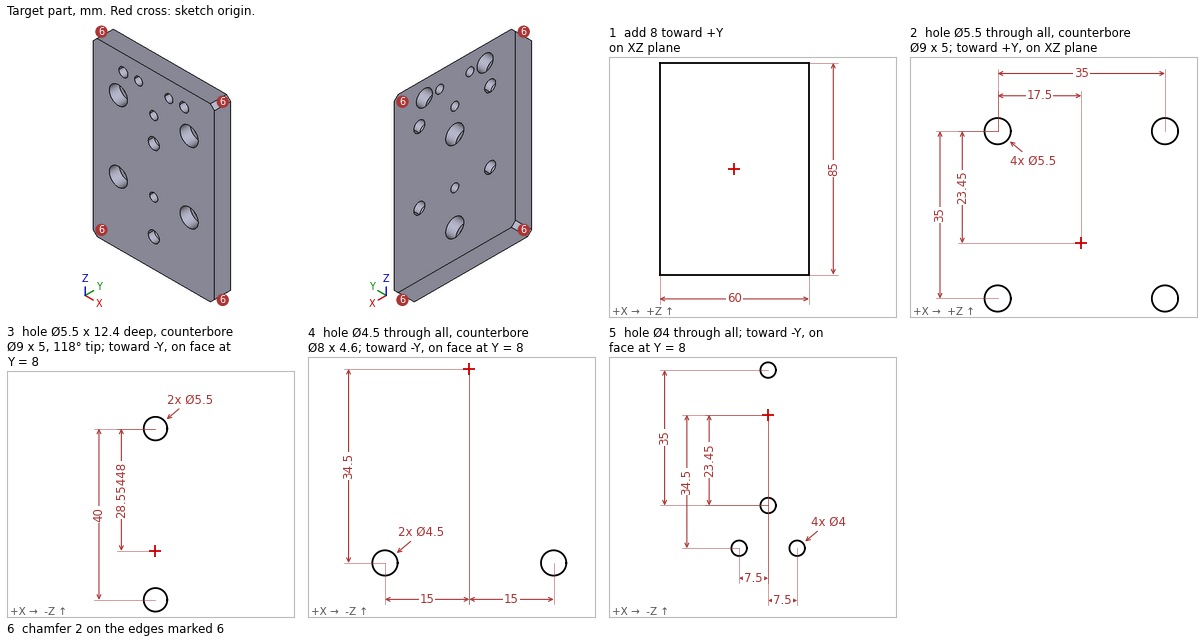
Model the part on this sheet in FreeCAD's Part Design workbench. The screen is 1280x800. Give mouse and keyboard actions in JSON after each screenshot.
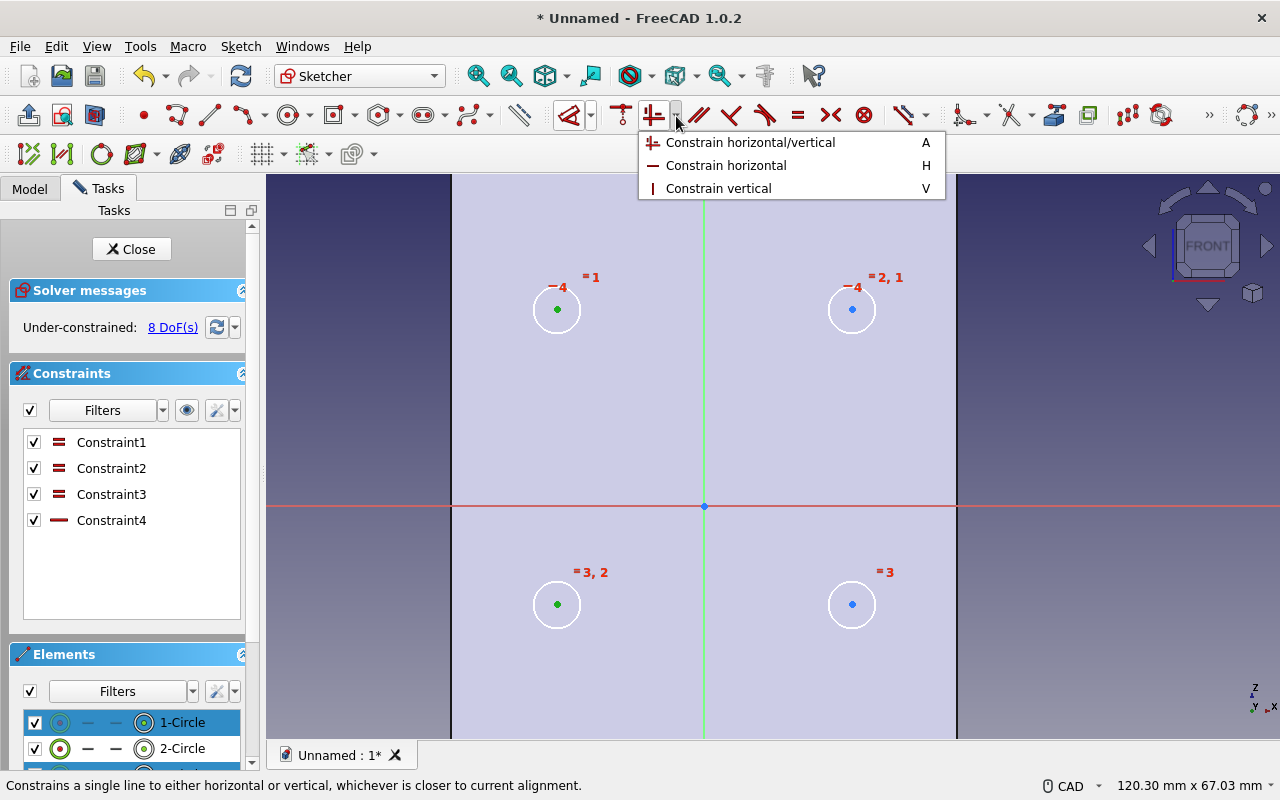
{"action": "left_click", "coordinate": [792, 188]}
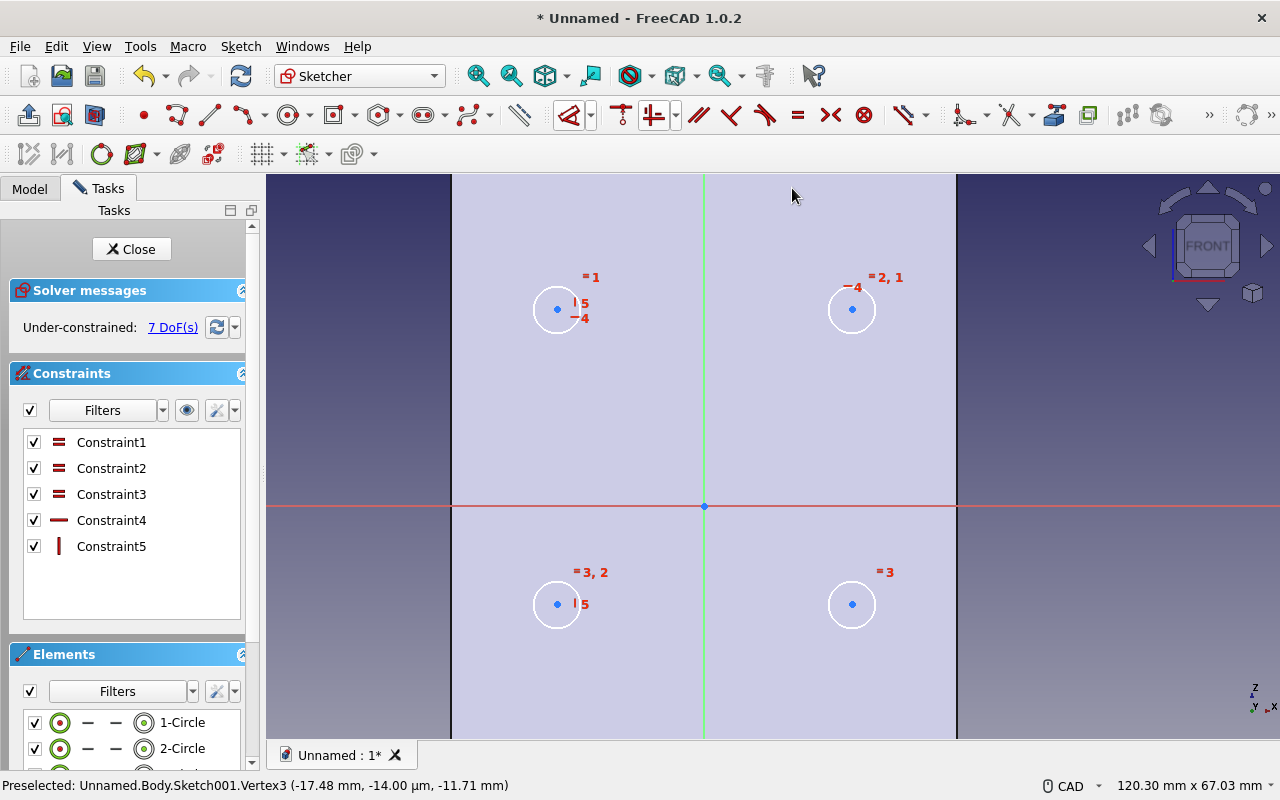
{"action": "left_click", "coordinate": [852, 310]}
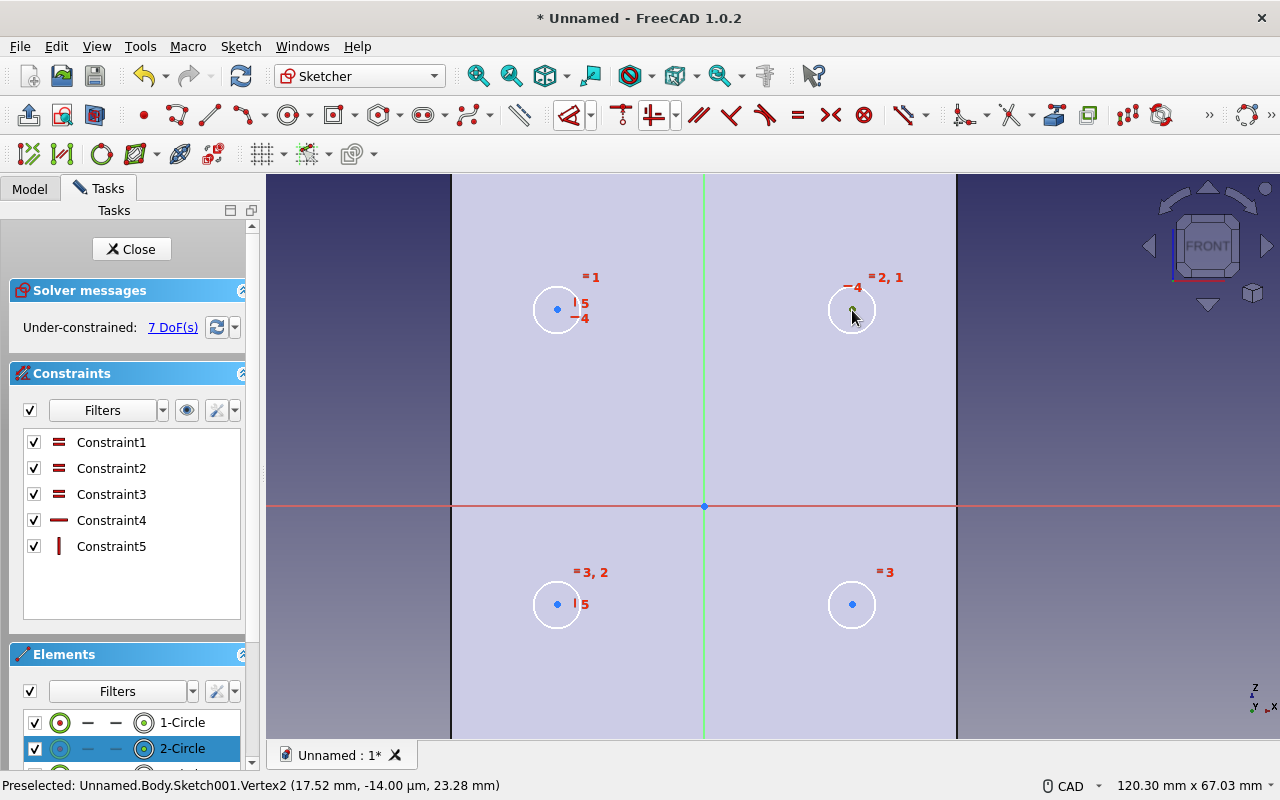
{"action": "left_click", "coordinate": [852, 605]}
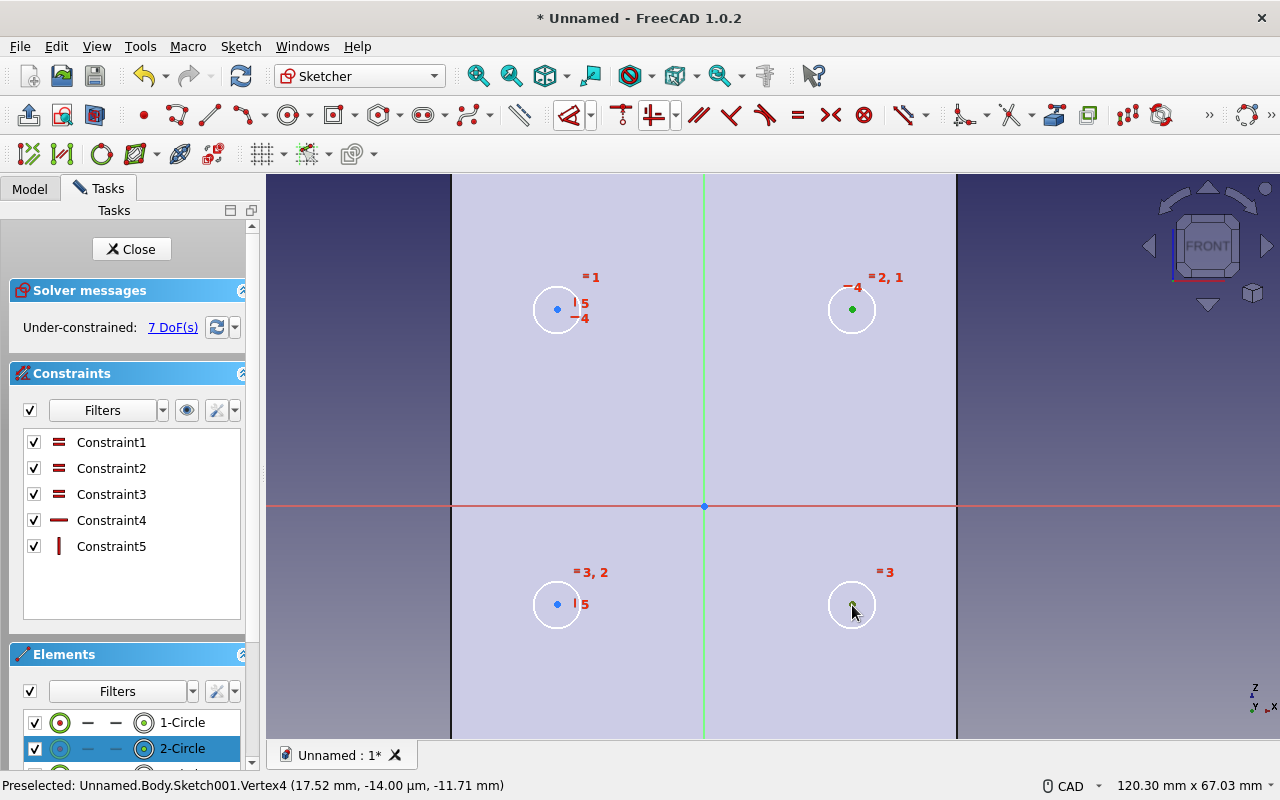
{"action": "key", "text": "v"}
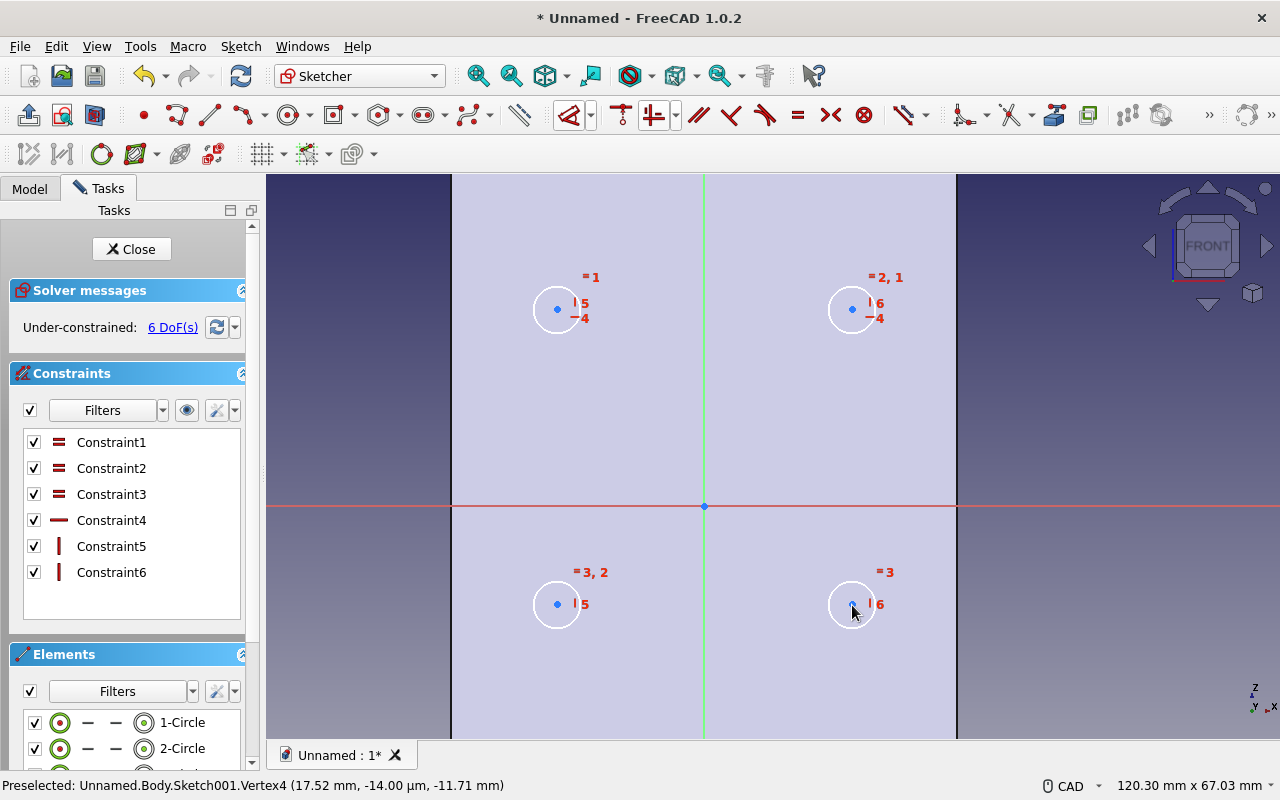
{"action": "left_click", "coordinate": [557, 605]}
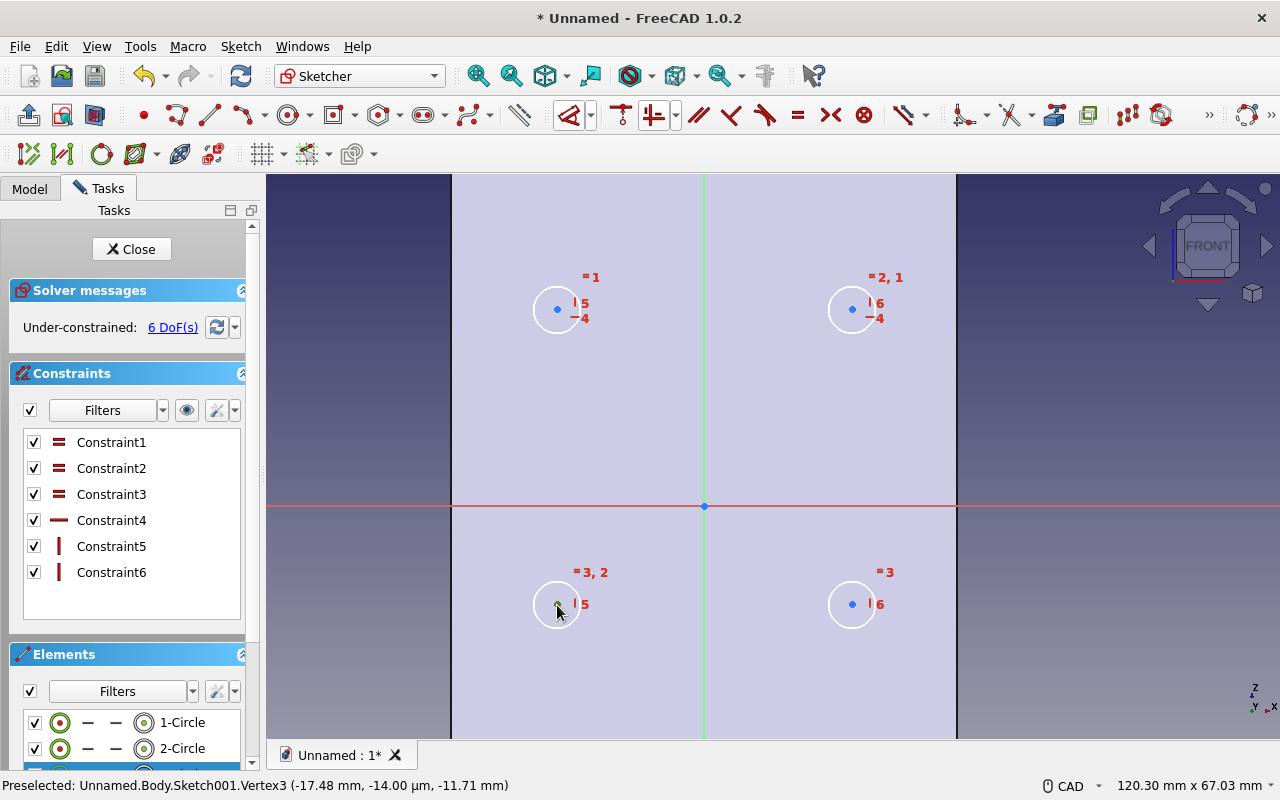
{"action": "left_click", "coordinate": [852, 605]}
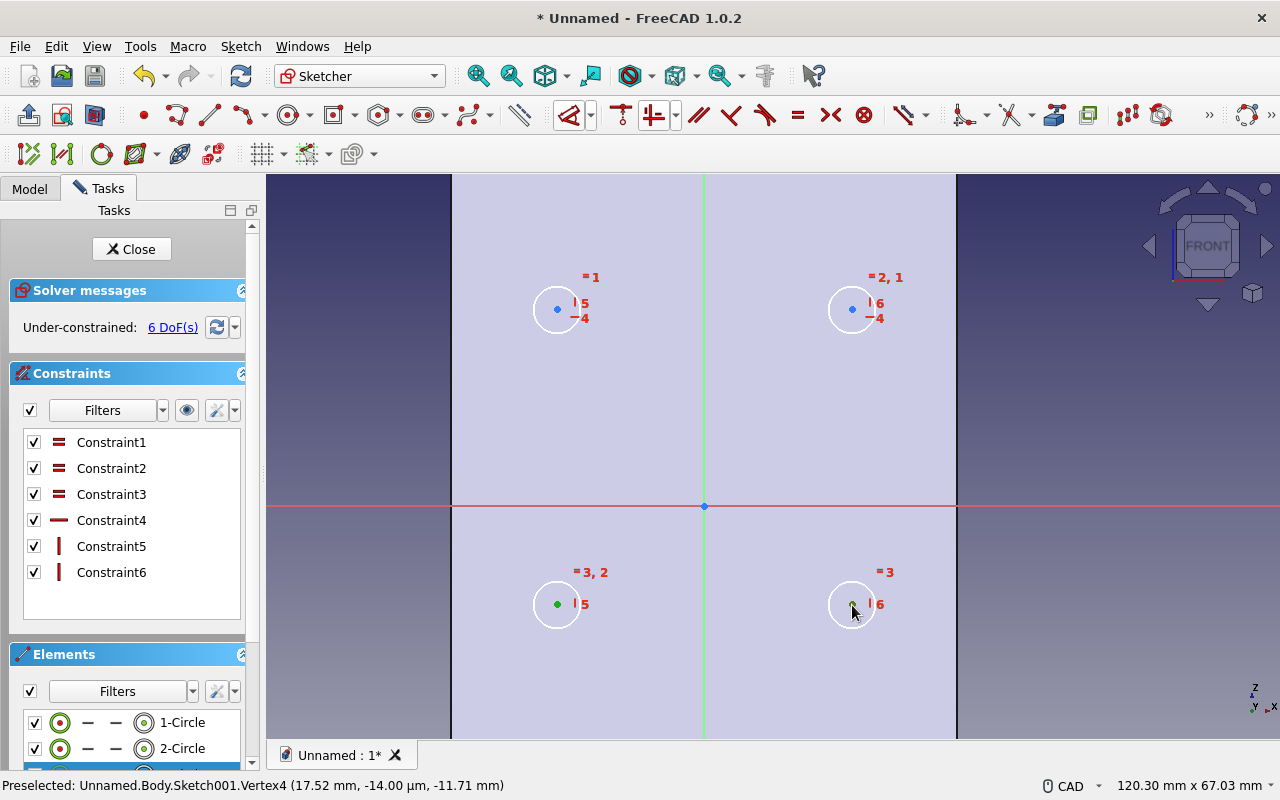
{"action": "key", "text": "h"}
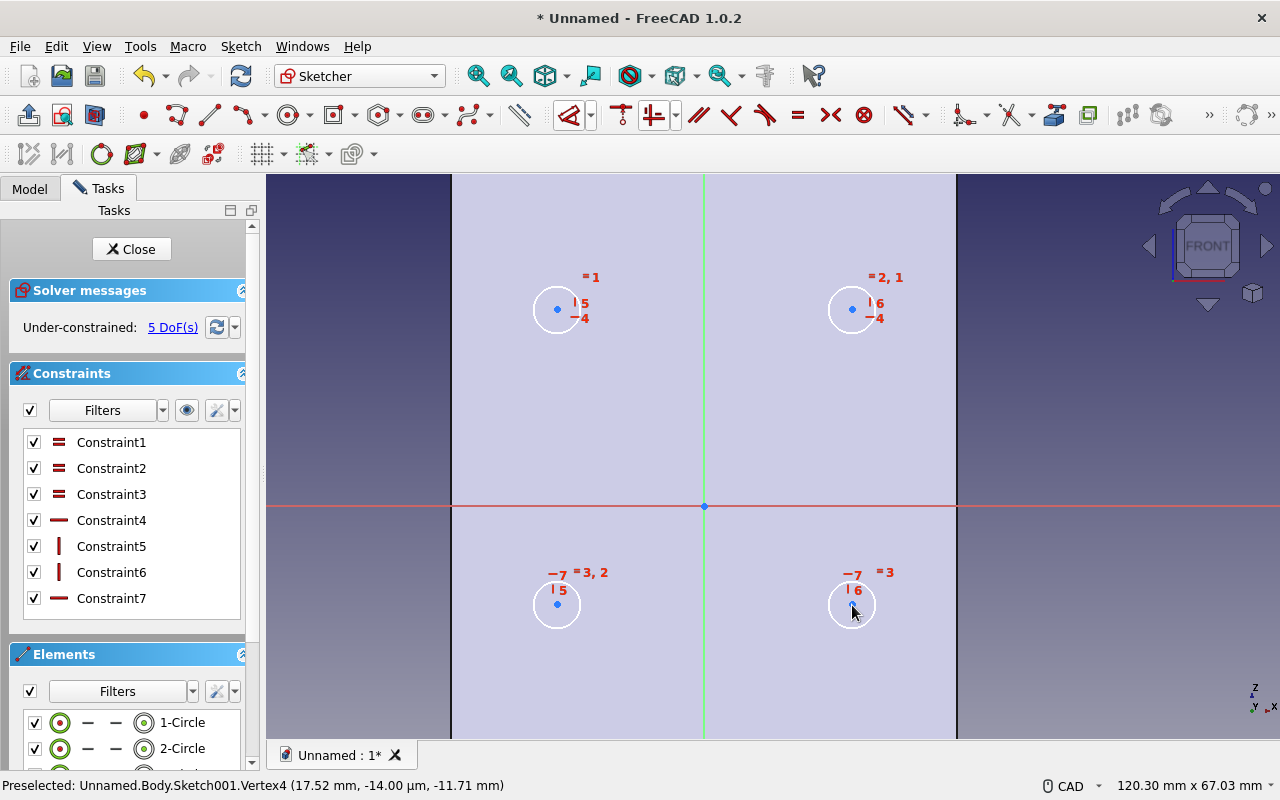
{"action": "left_click", "coordinate": [573, 293]}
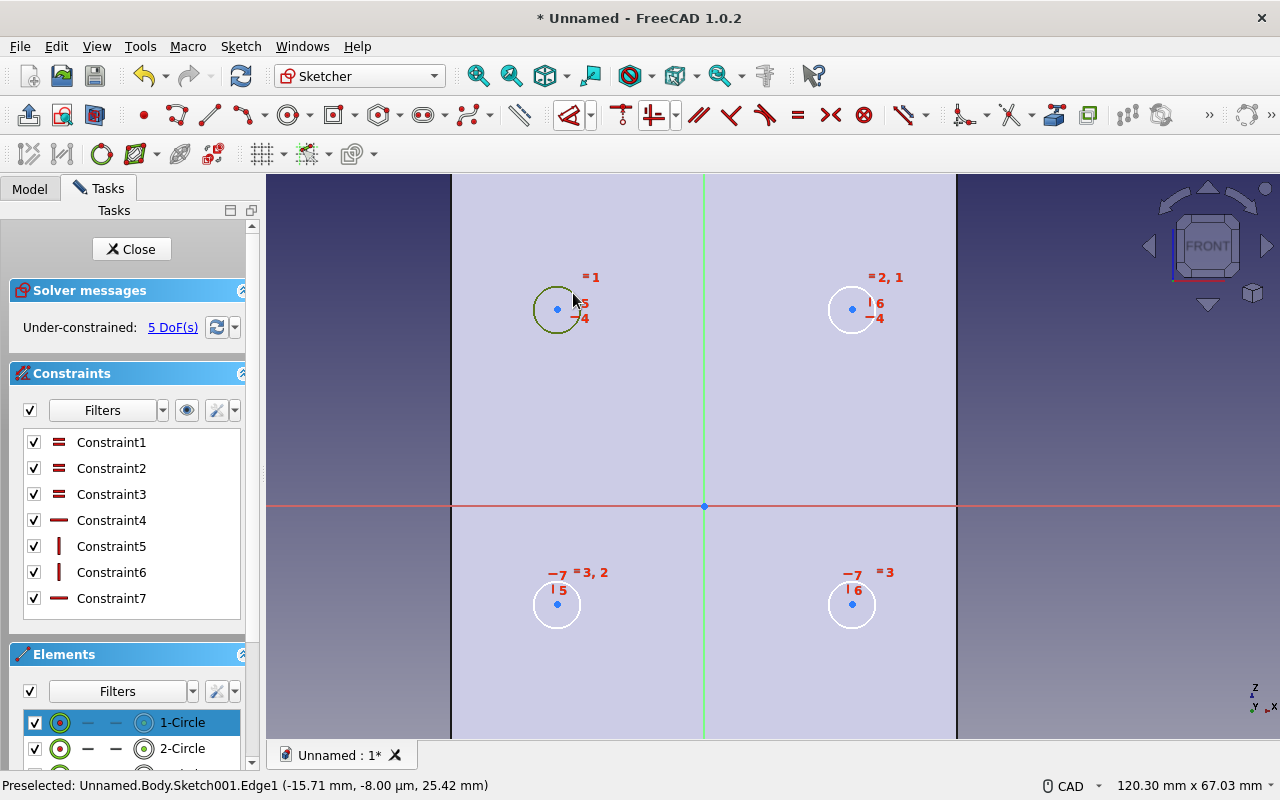
{"action": "left_click", "coordinate": [590, 116]}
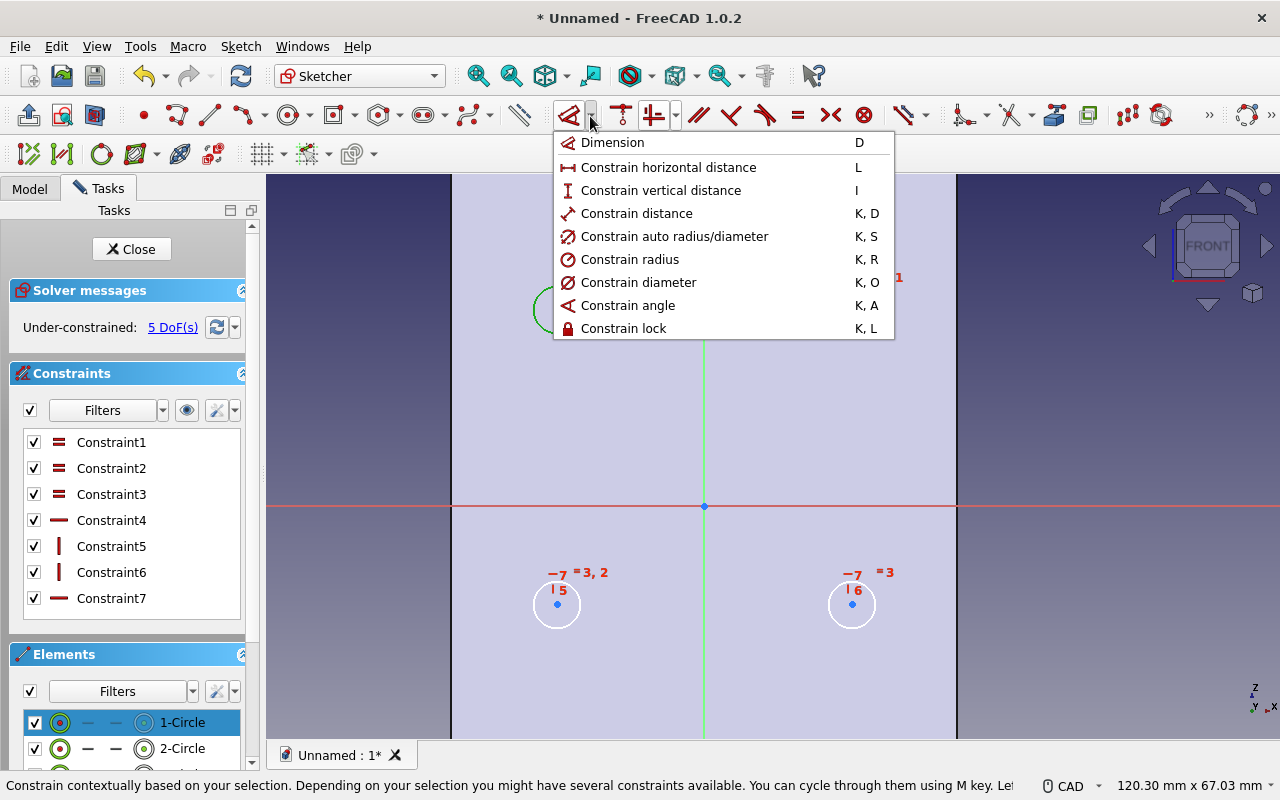
{"action": "left_click", "coordinate": [724, 282]}